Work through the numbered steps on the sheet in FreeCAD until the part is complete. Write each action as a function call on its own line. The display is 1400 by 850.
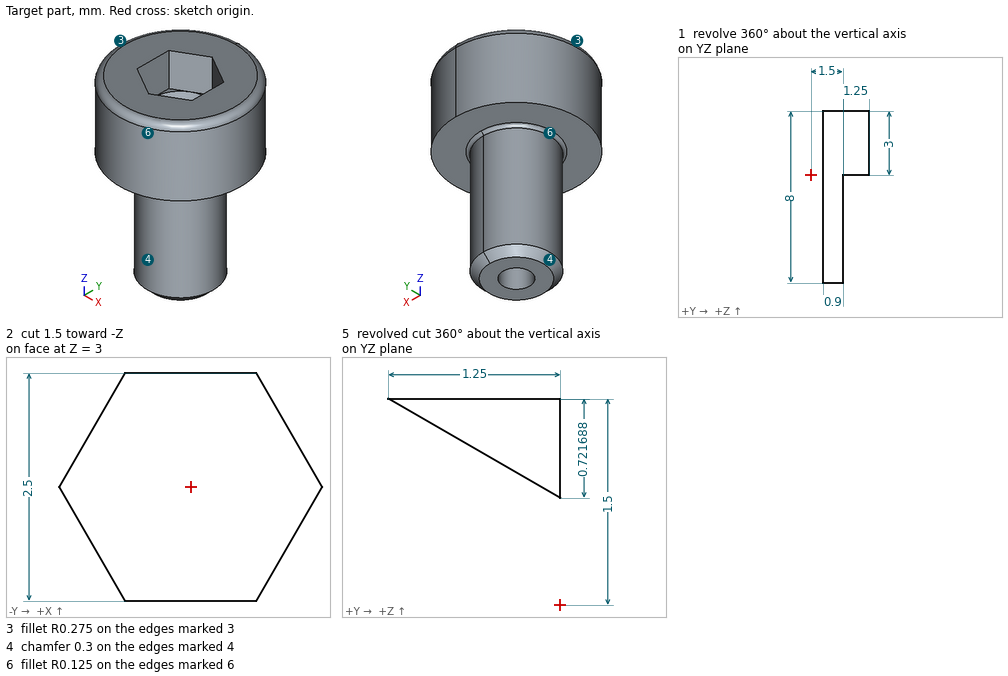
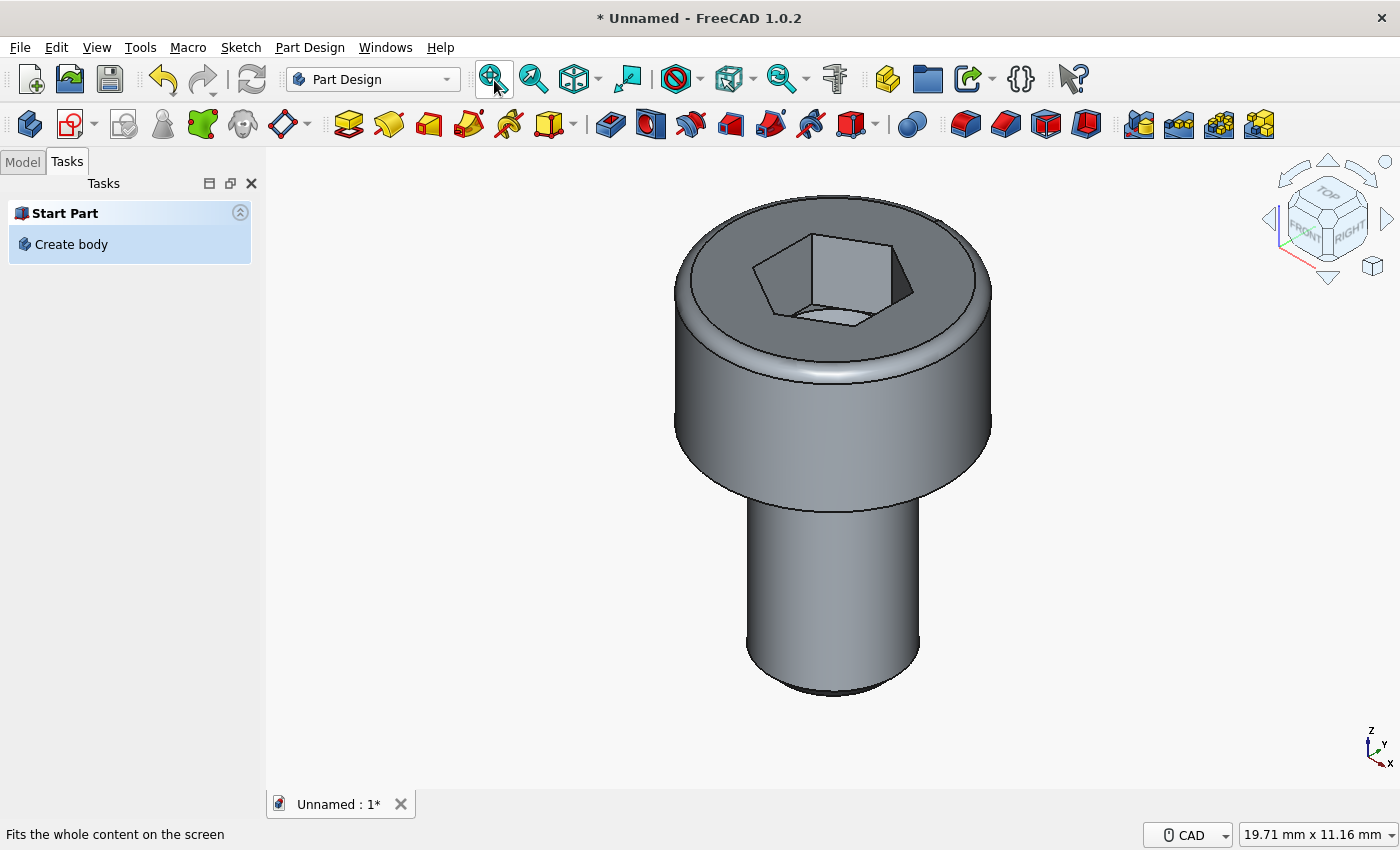
key(2)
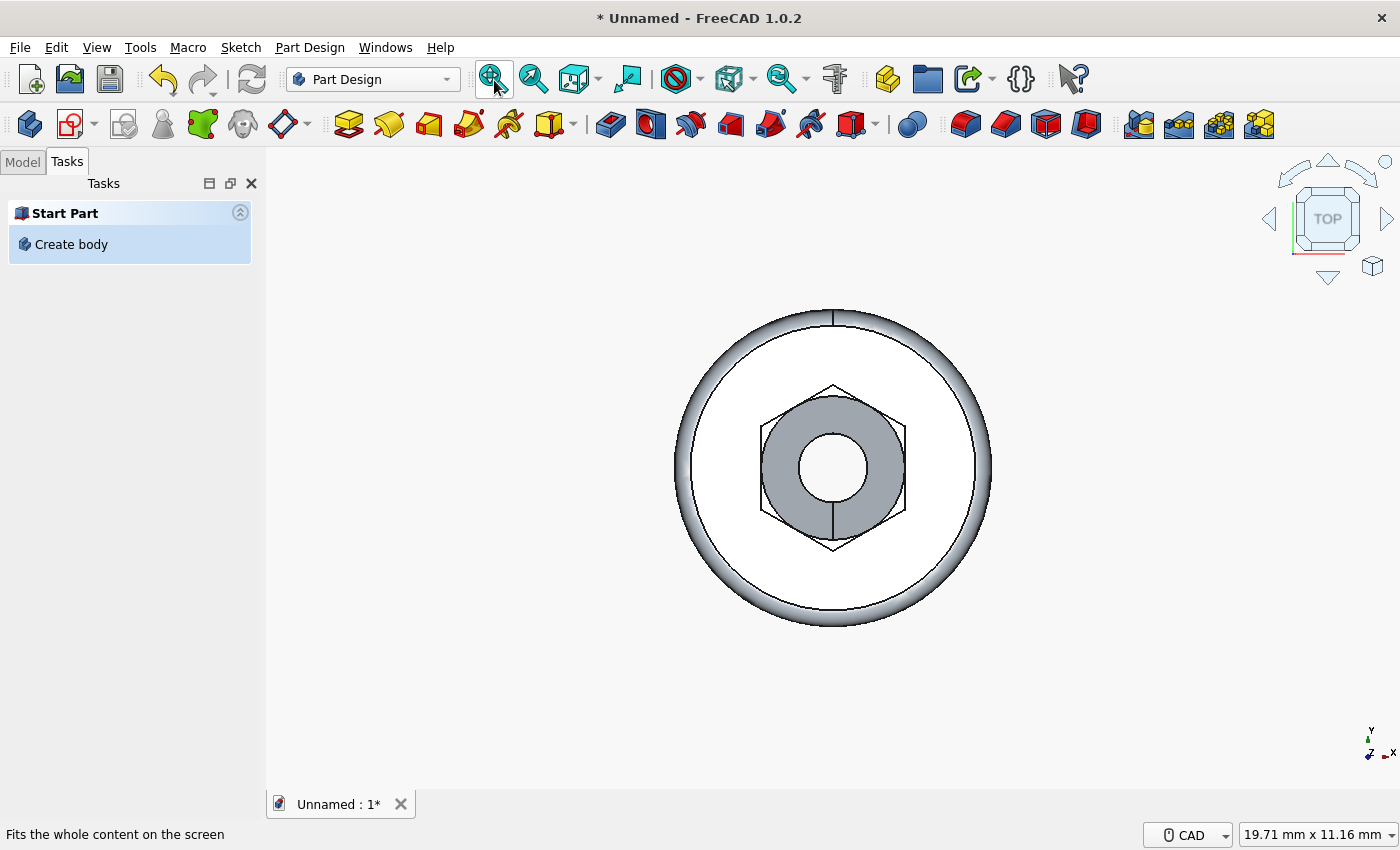
key(1)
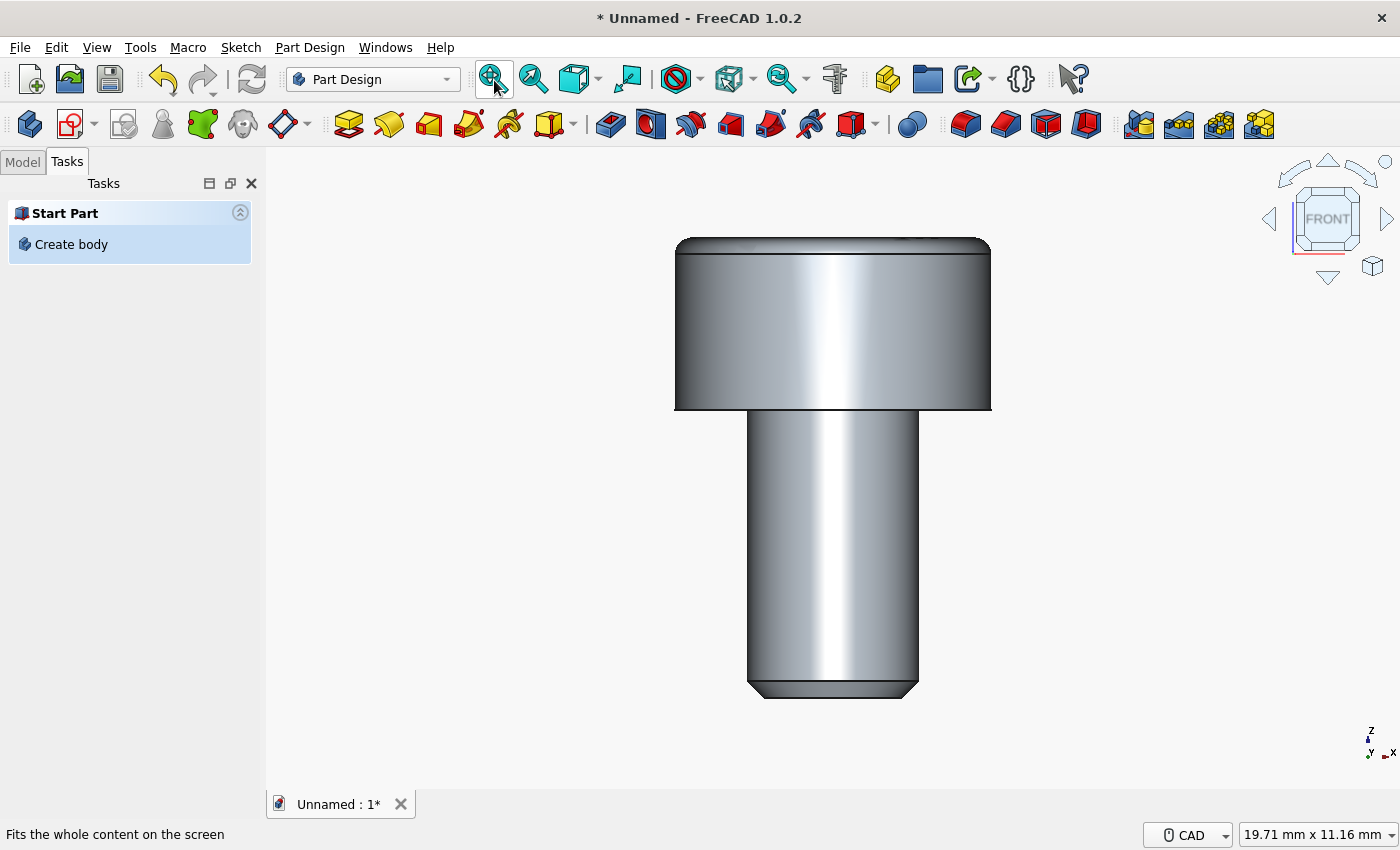
key(3)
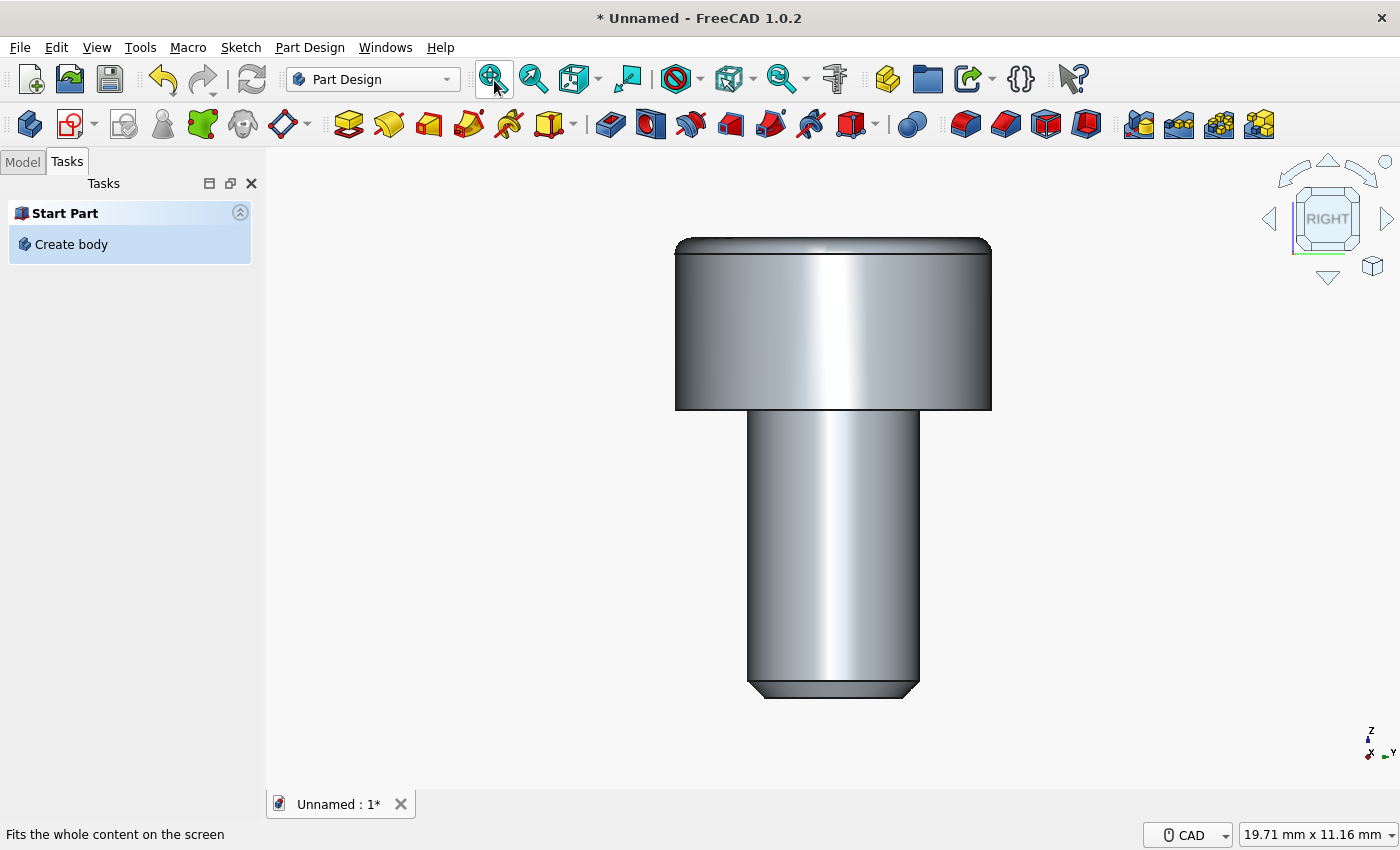
key(5)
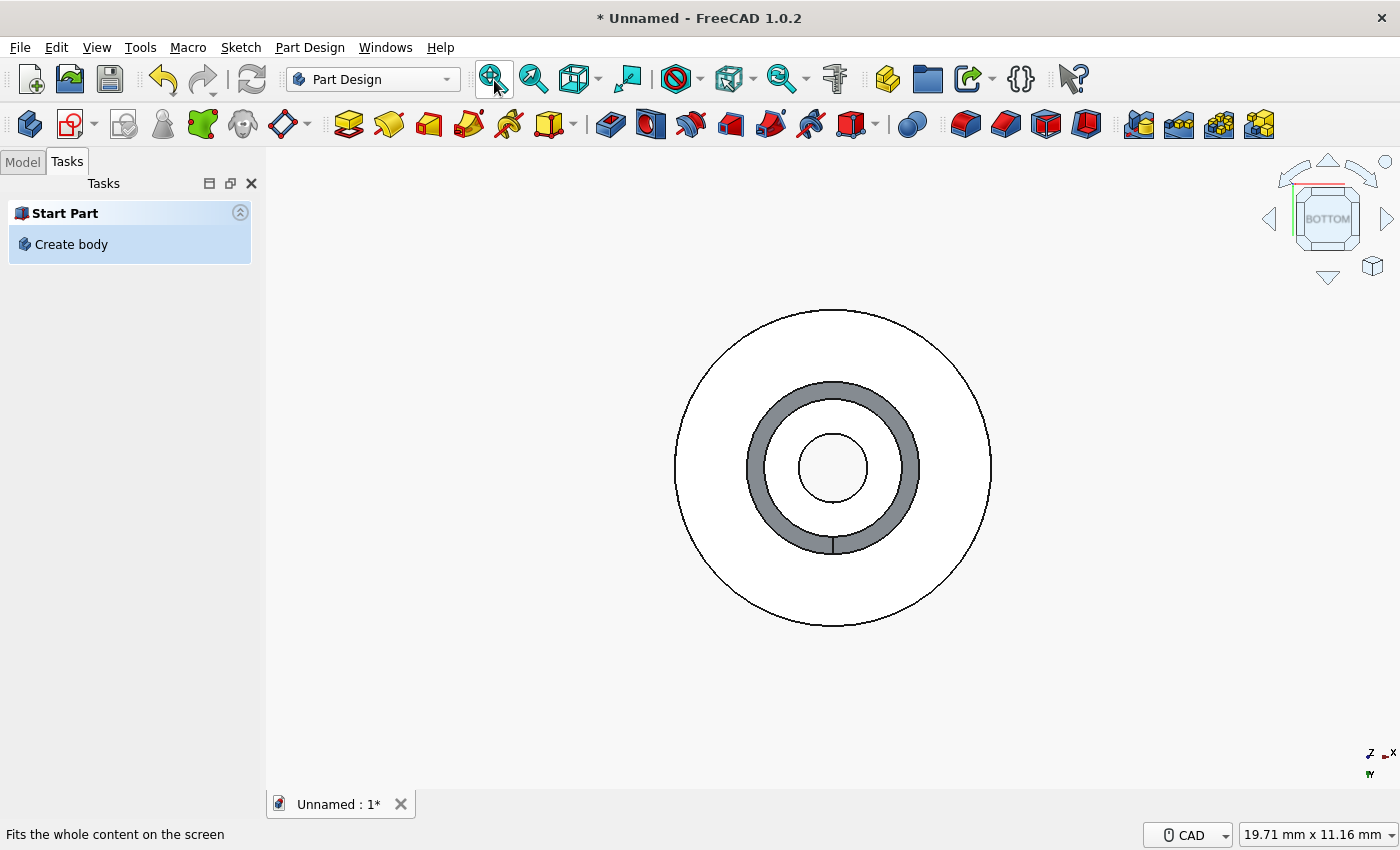
key(4)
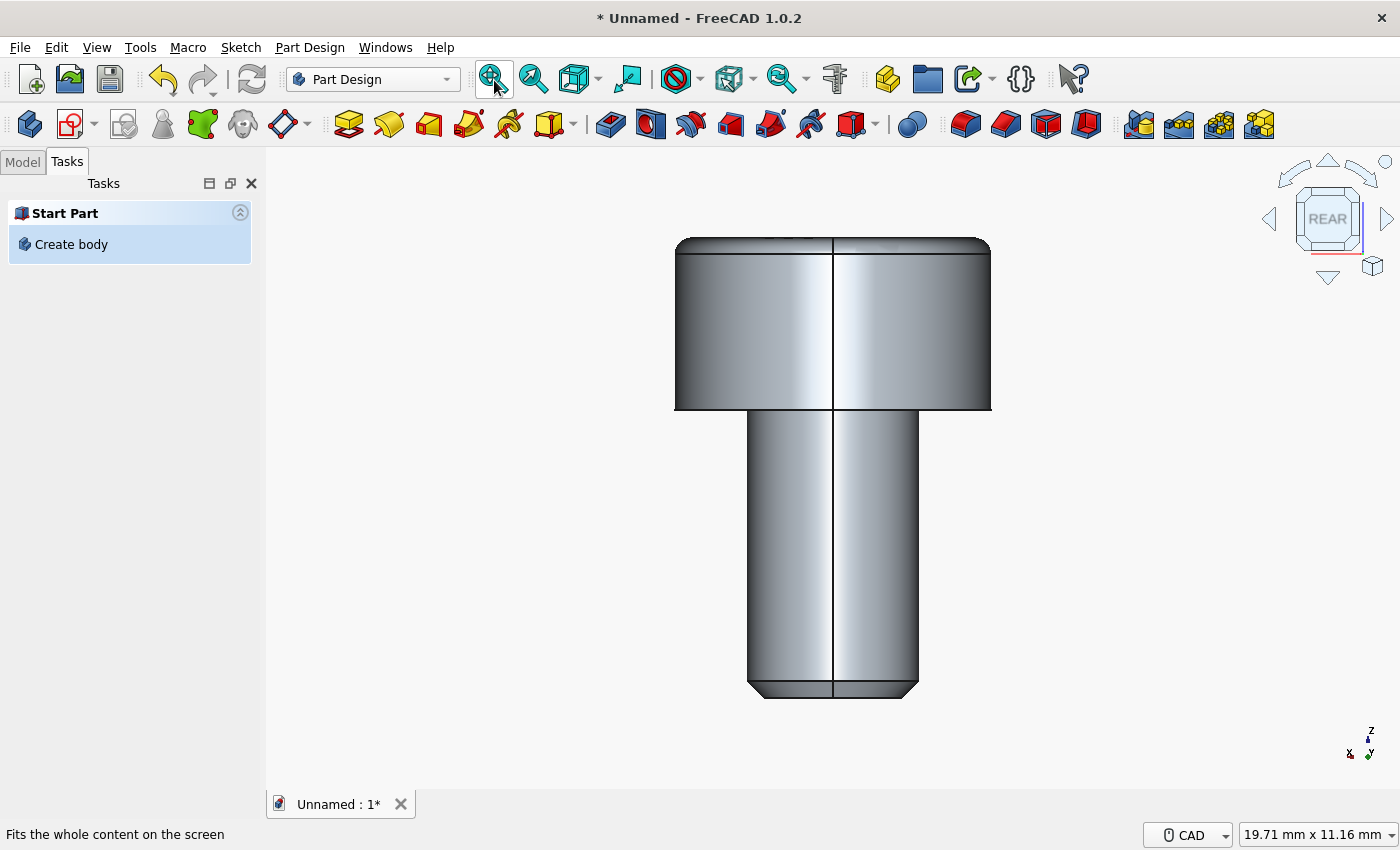
key(6)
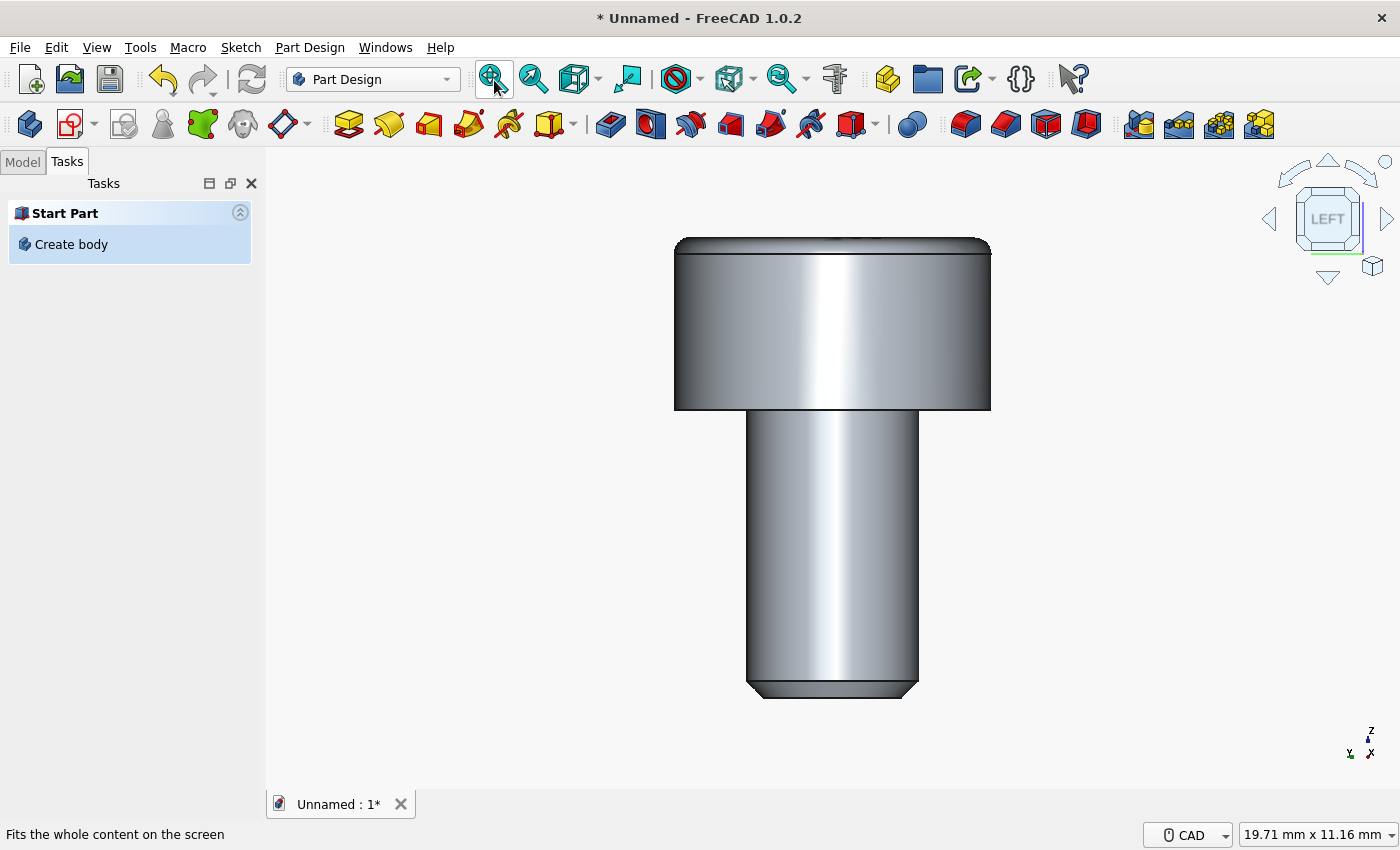
key(v)
key(3)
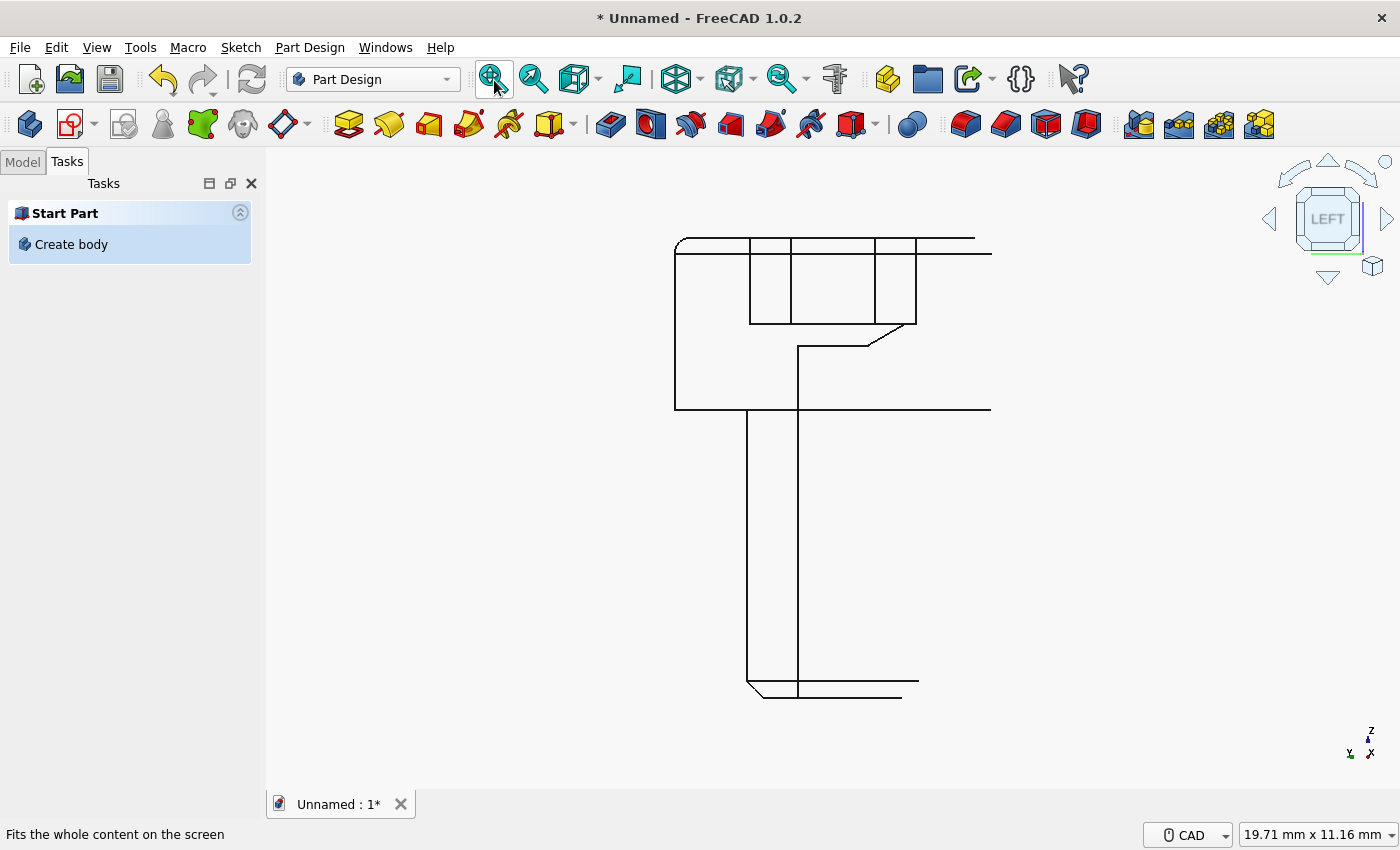
key(0)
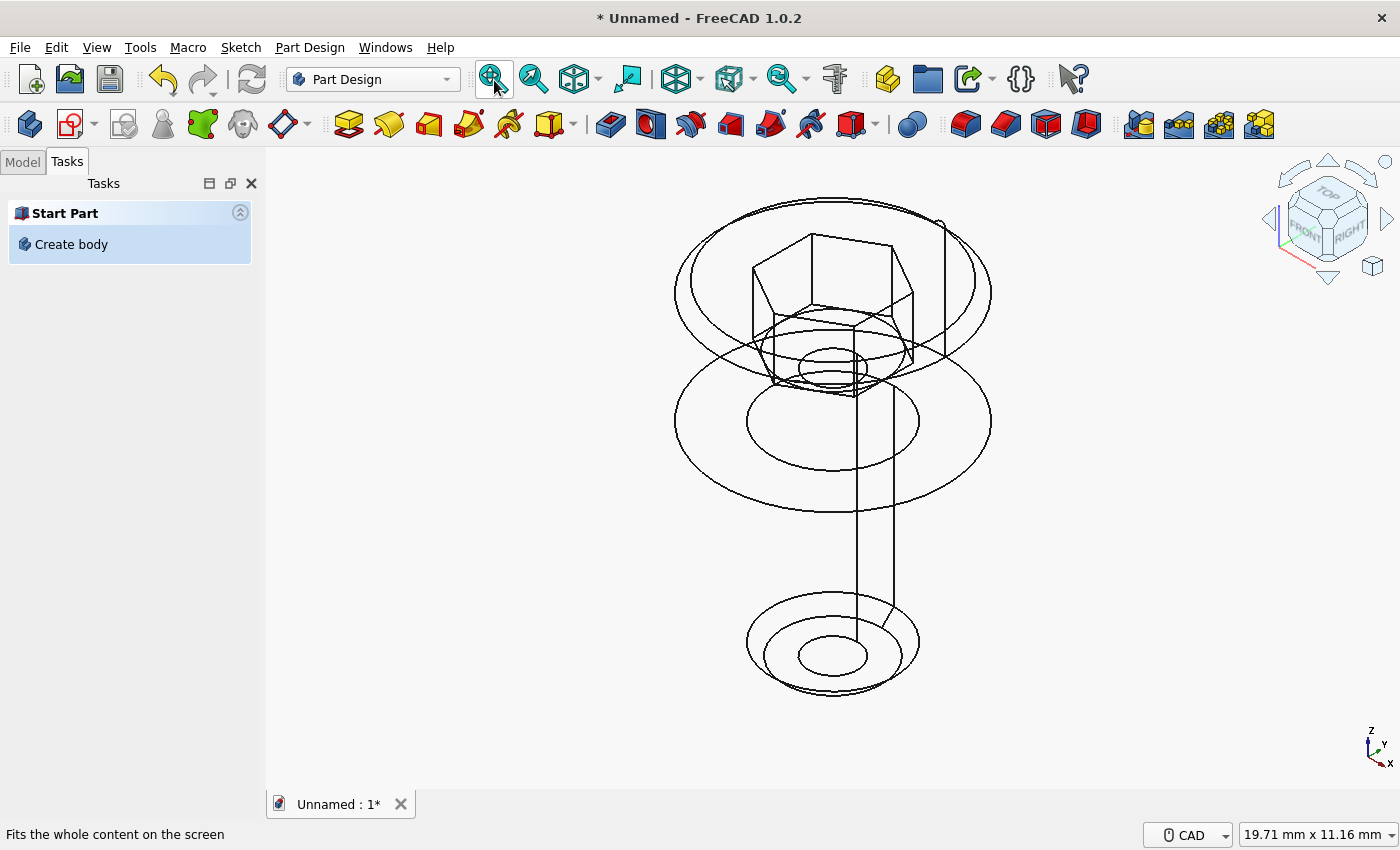
click(772, 455)